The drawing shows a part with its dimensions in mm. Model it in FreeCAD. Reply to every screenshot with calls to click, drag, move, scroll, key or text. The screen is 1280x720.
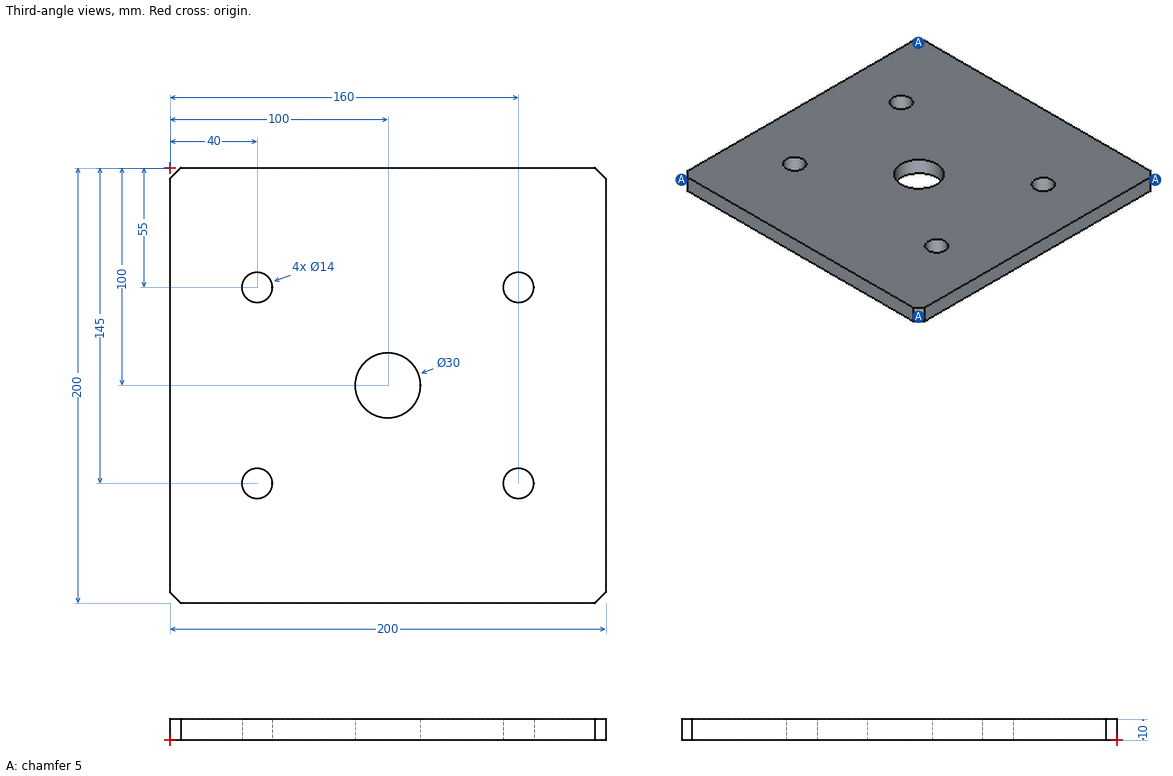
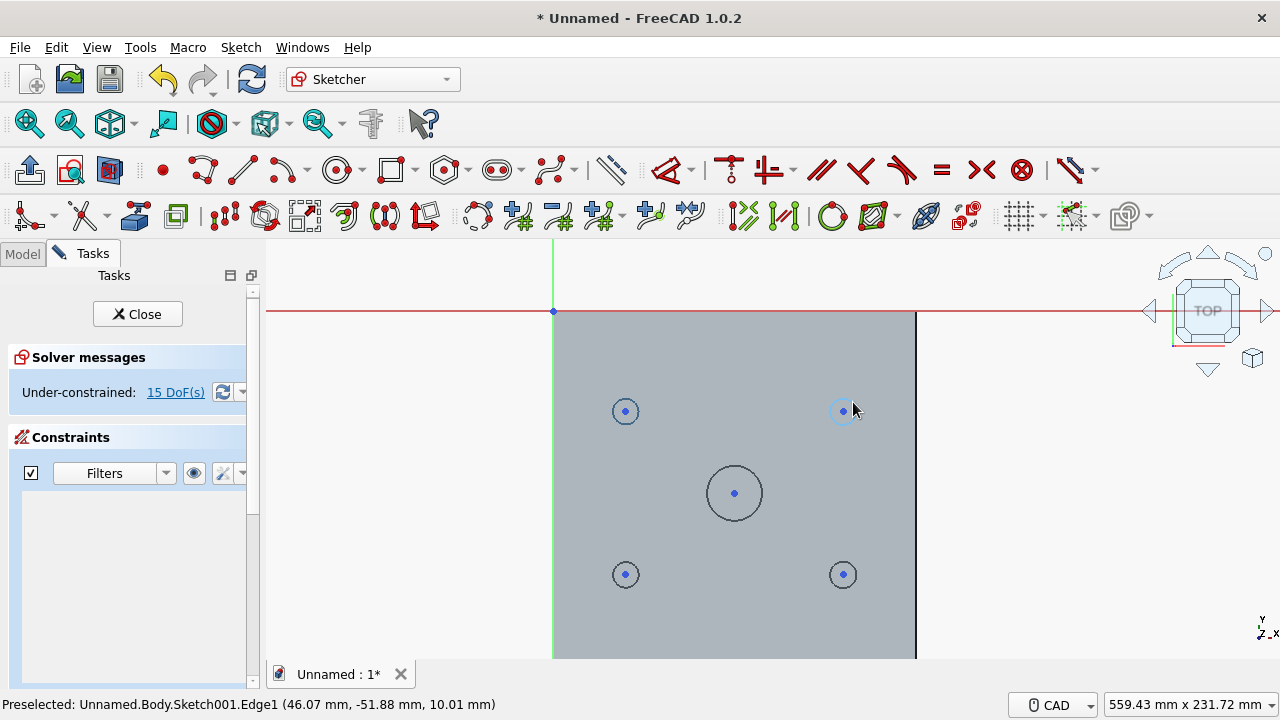
click(635, 566)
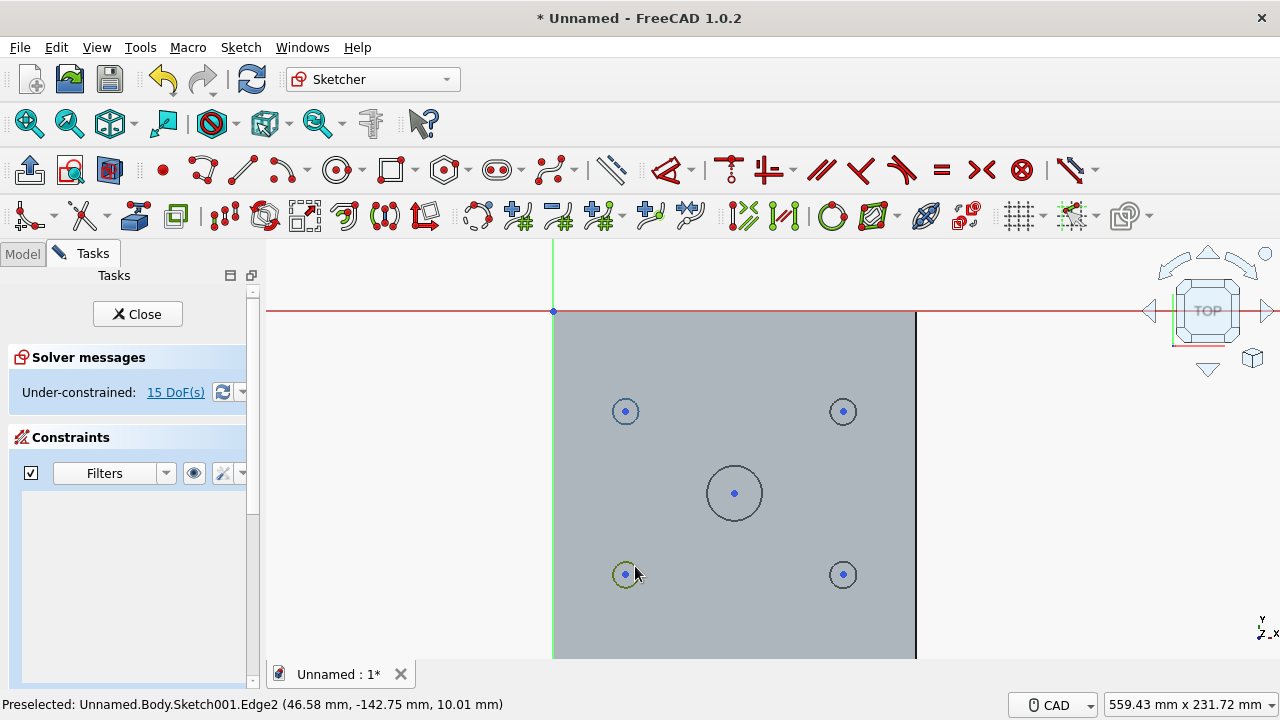
click(853, 566)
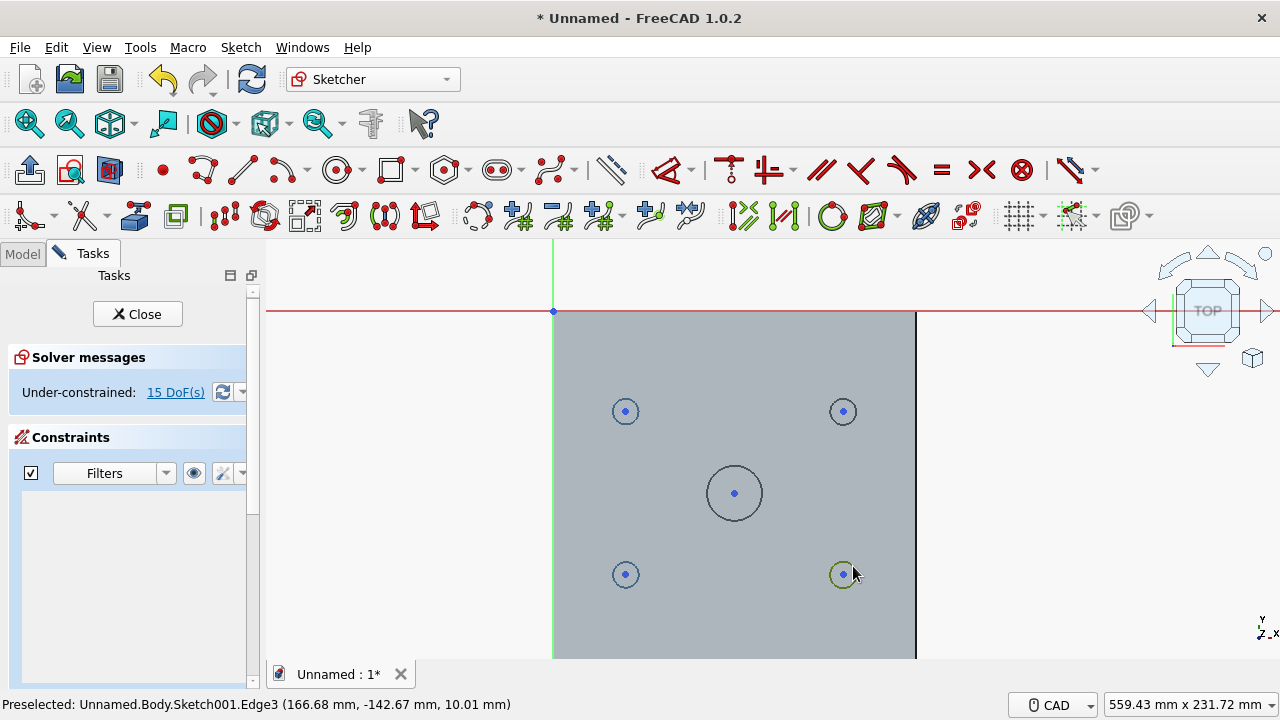
click(852, 403)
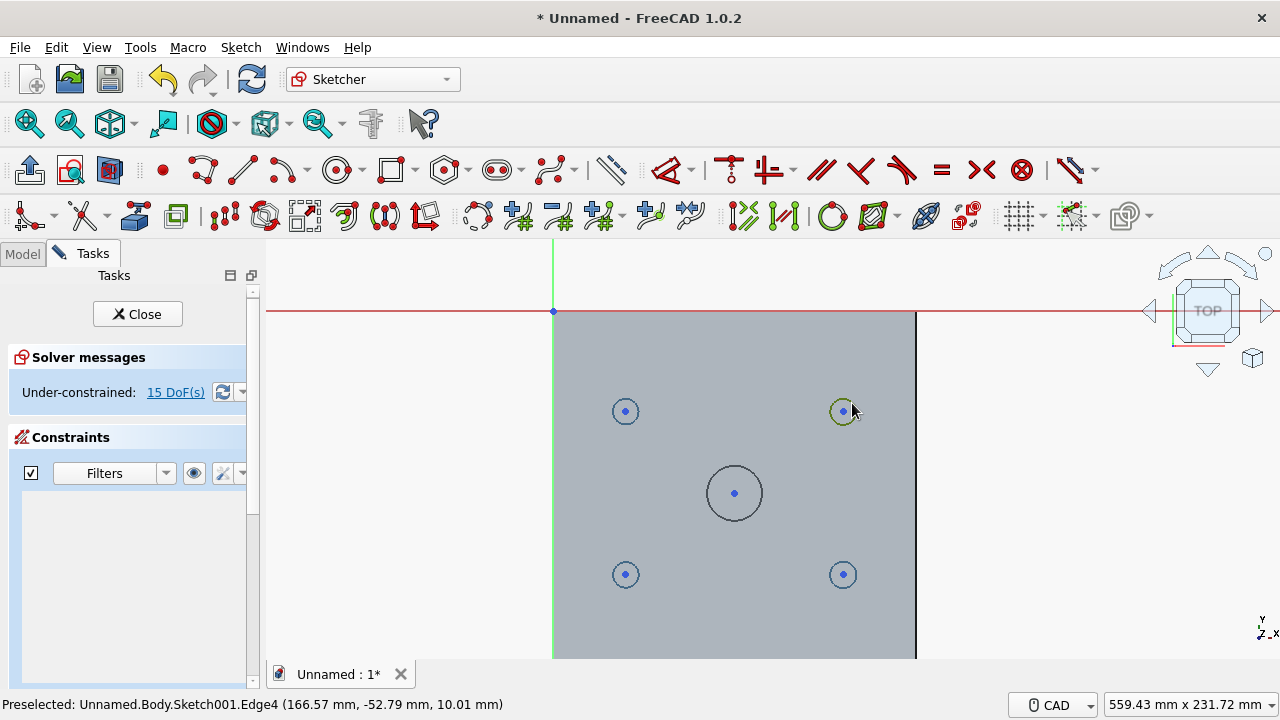
click(942, 170)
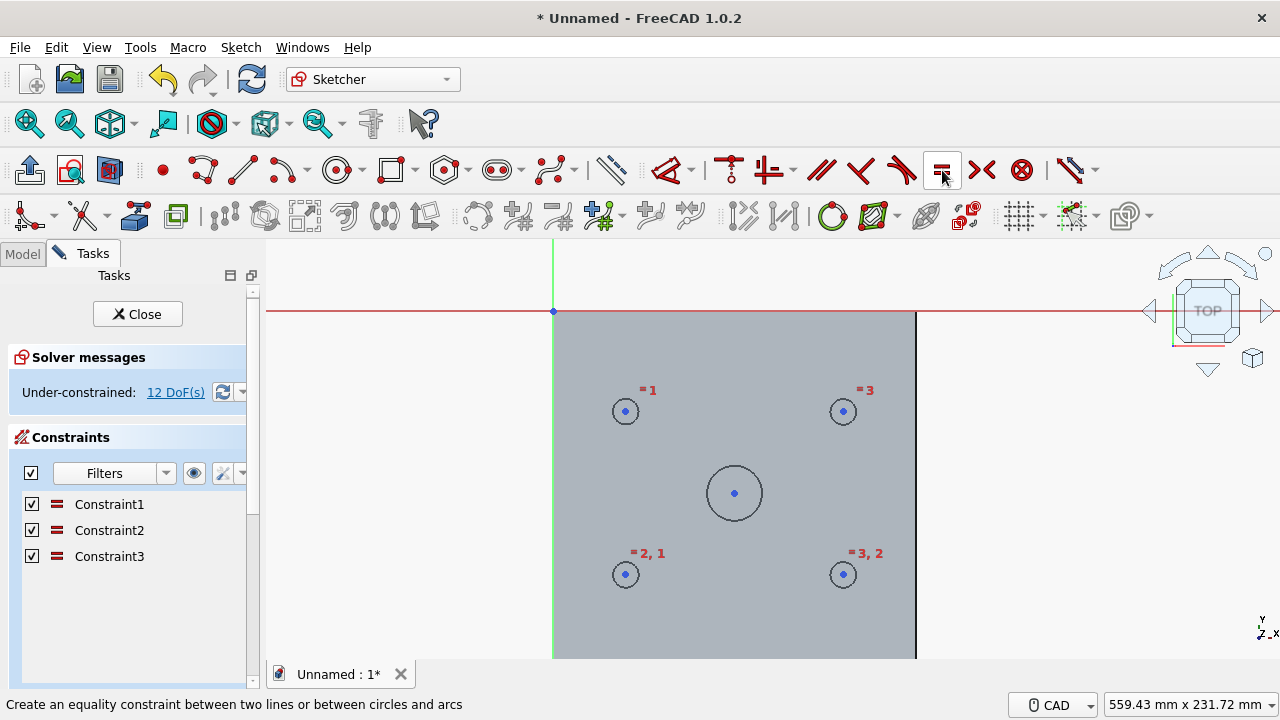
click(626, 412)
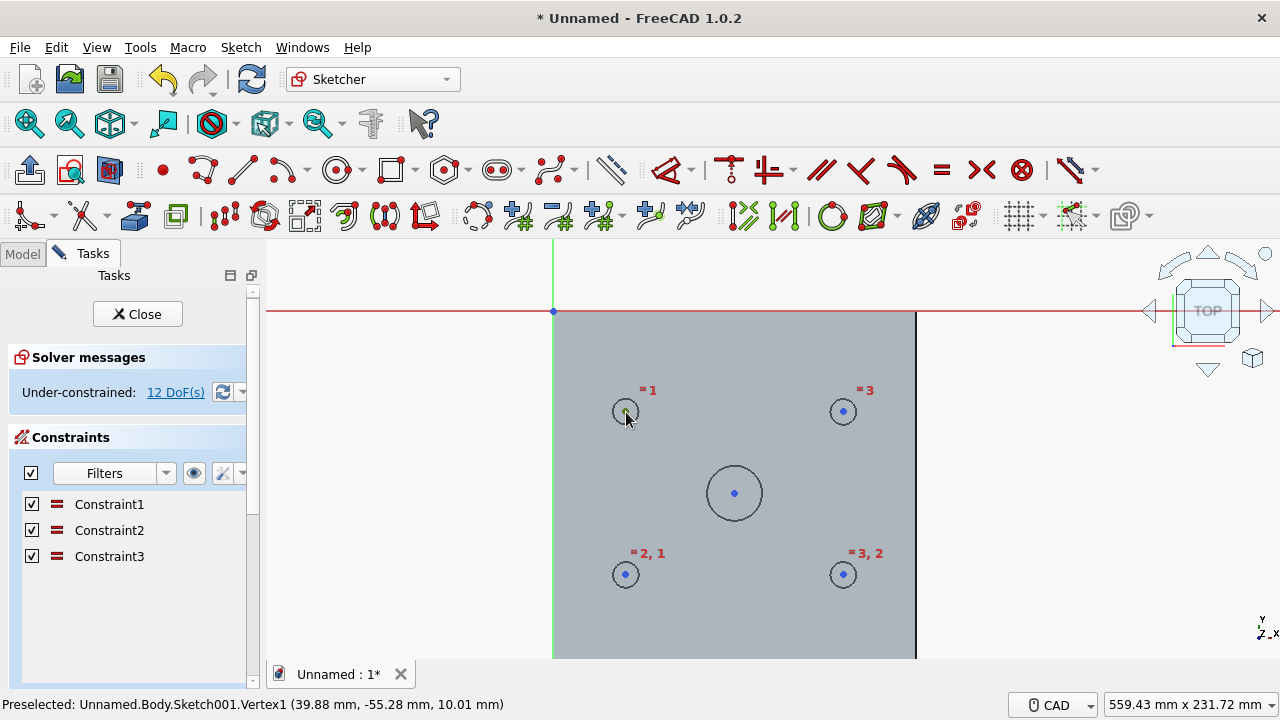
click(626, 575)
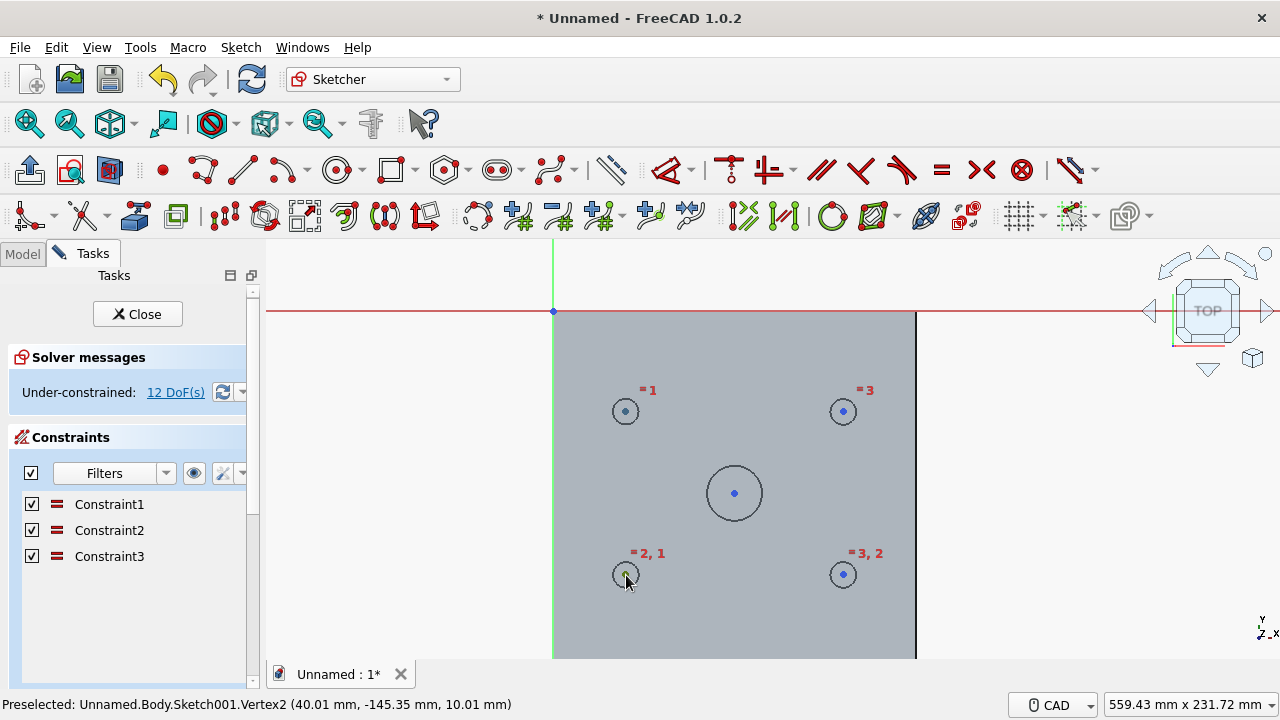
click(796, 170)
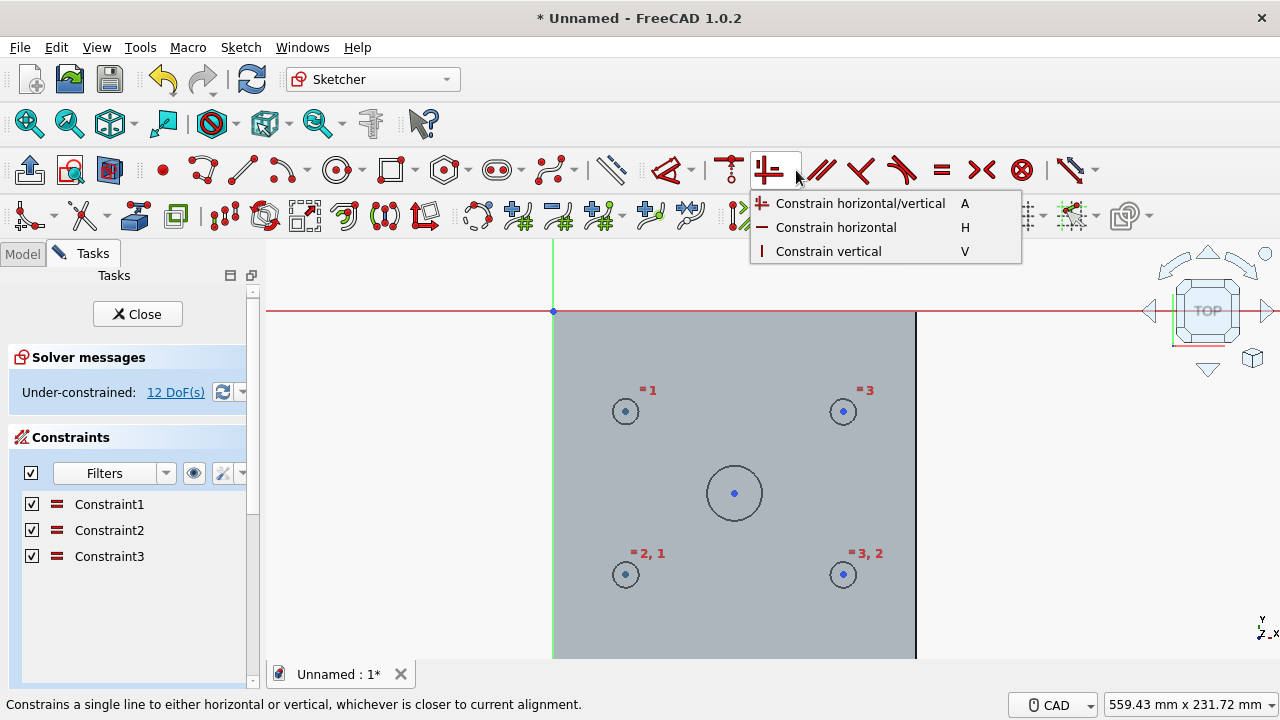
click(886, 251)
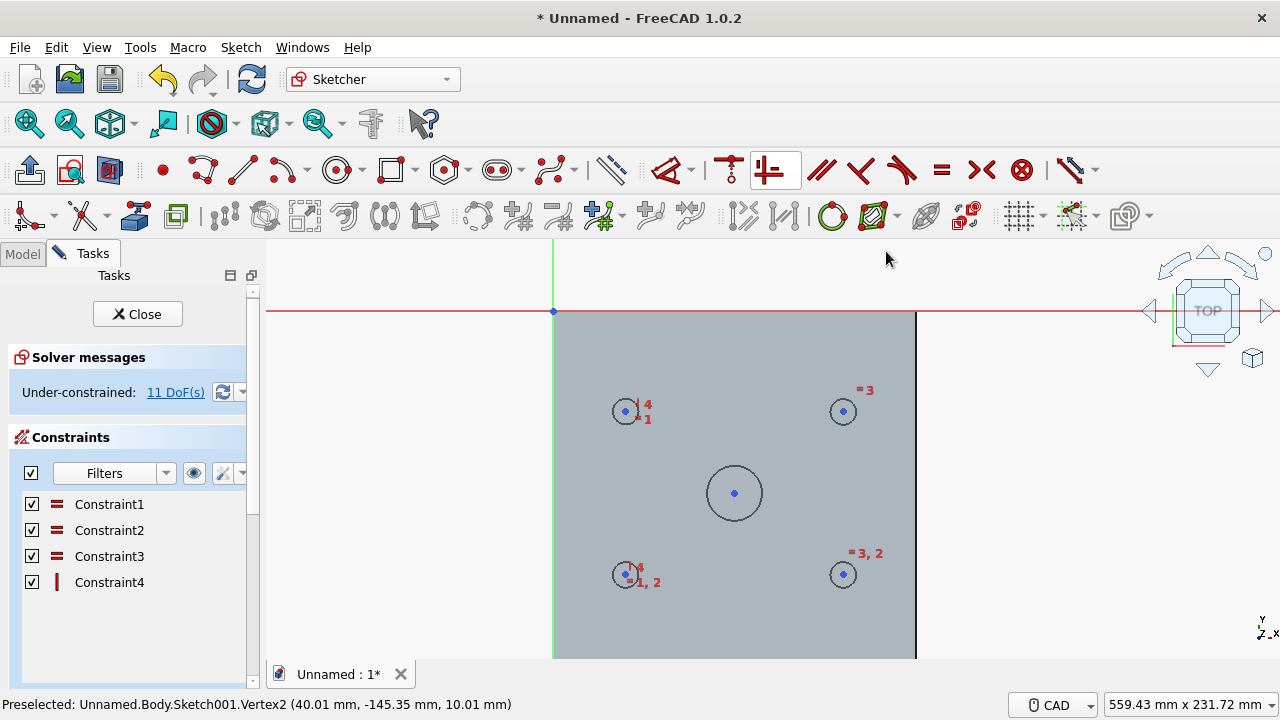
click(624, 577)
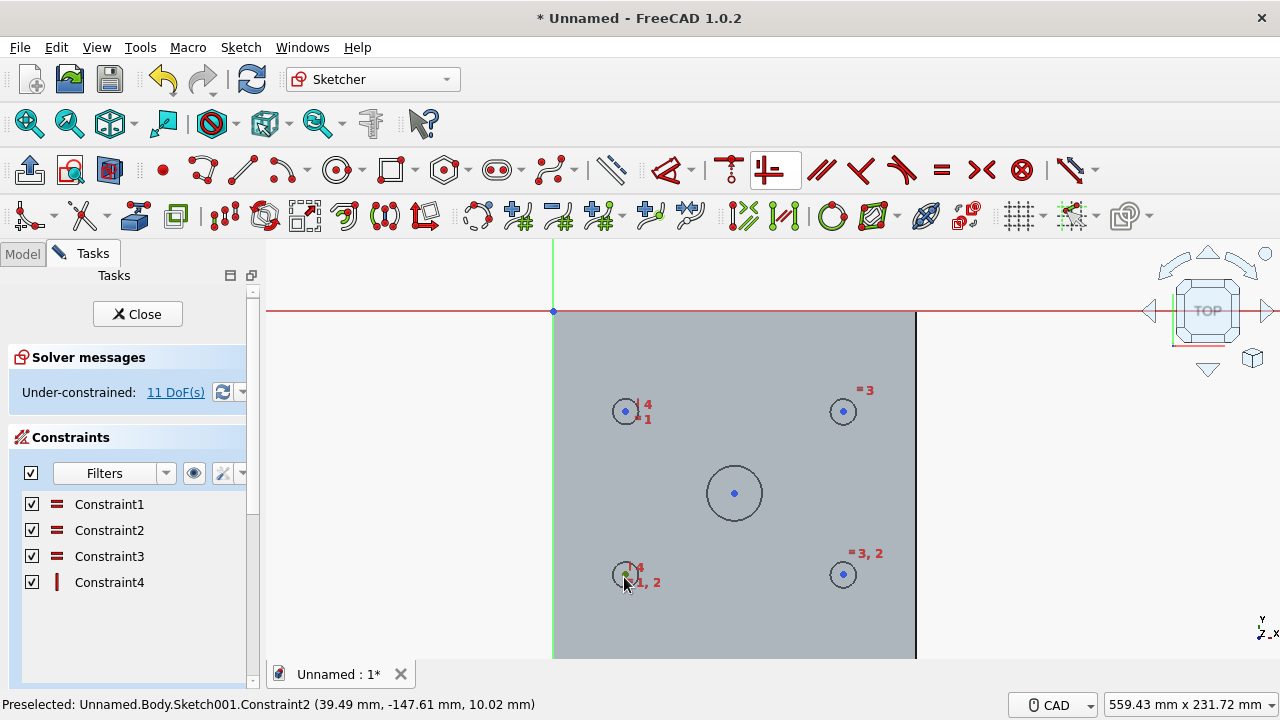
click(843, 575)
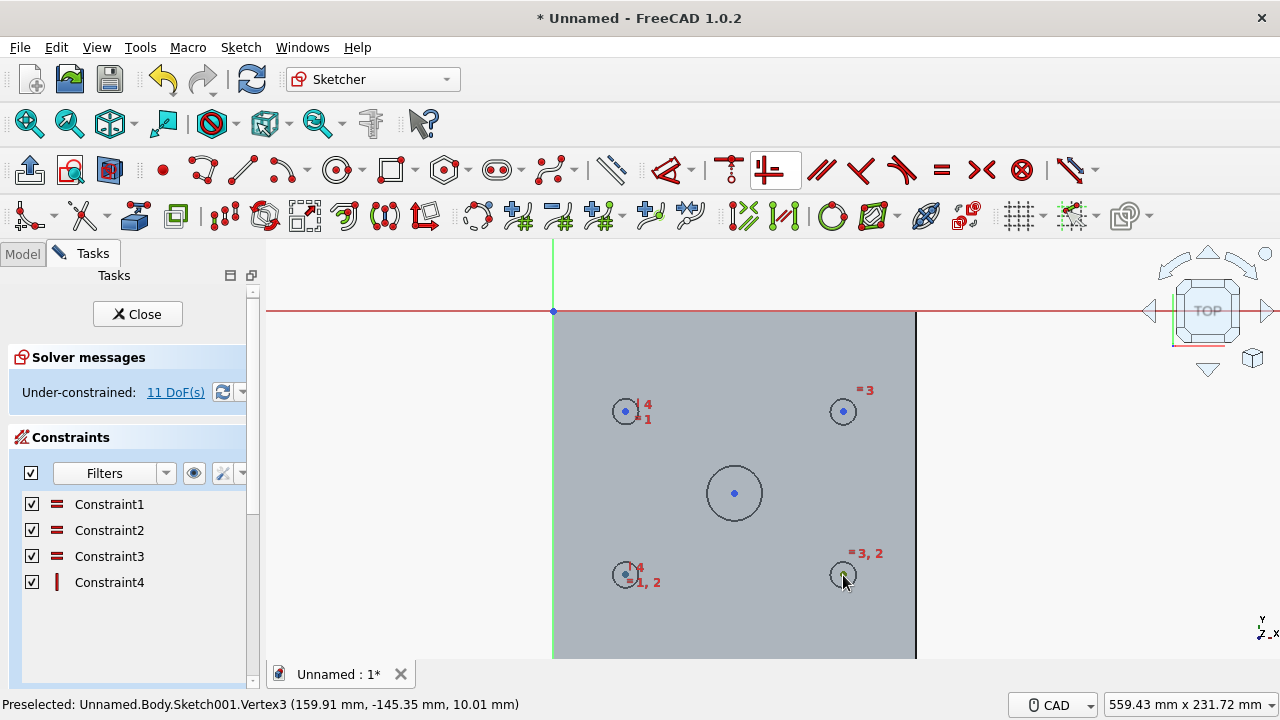
click(796, 170)